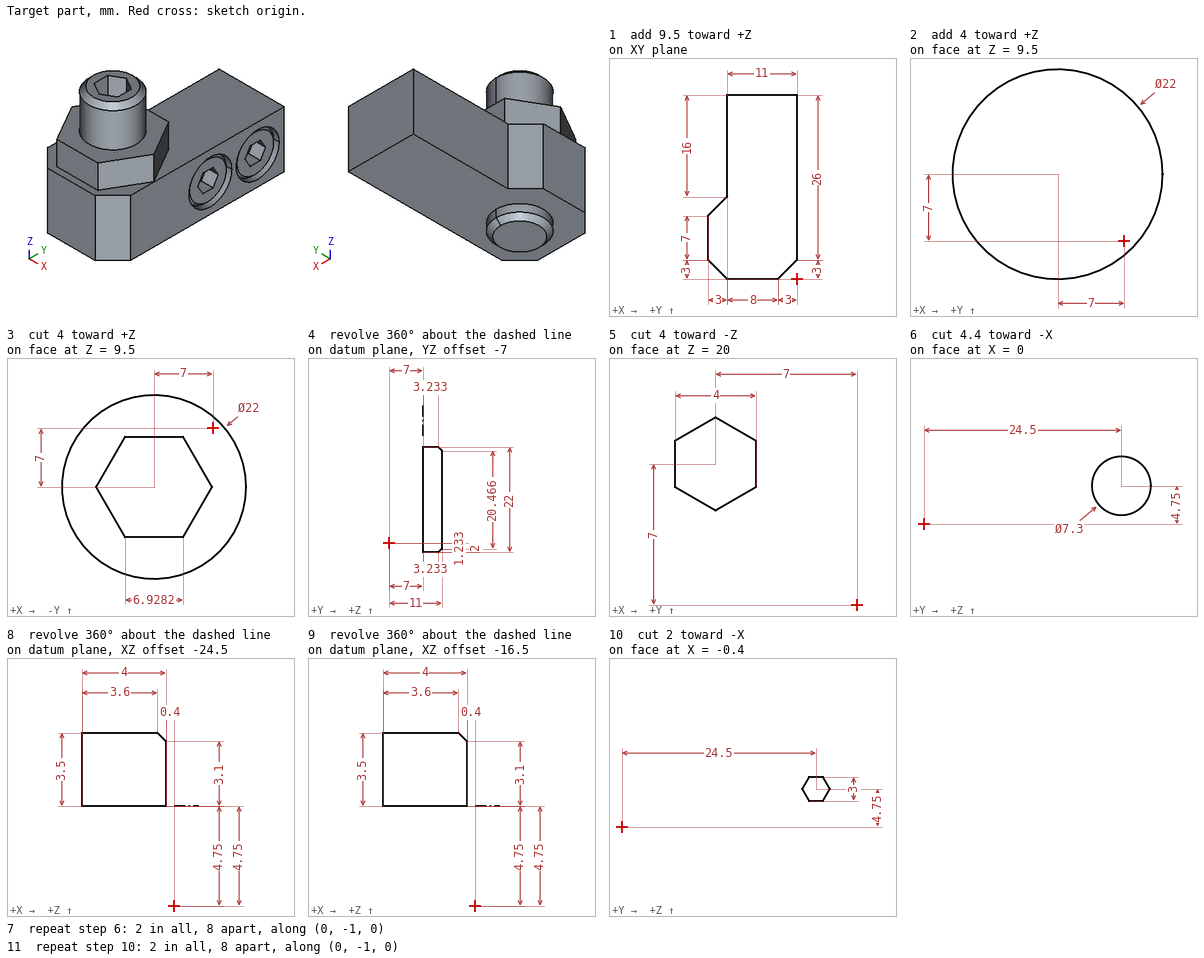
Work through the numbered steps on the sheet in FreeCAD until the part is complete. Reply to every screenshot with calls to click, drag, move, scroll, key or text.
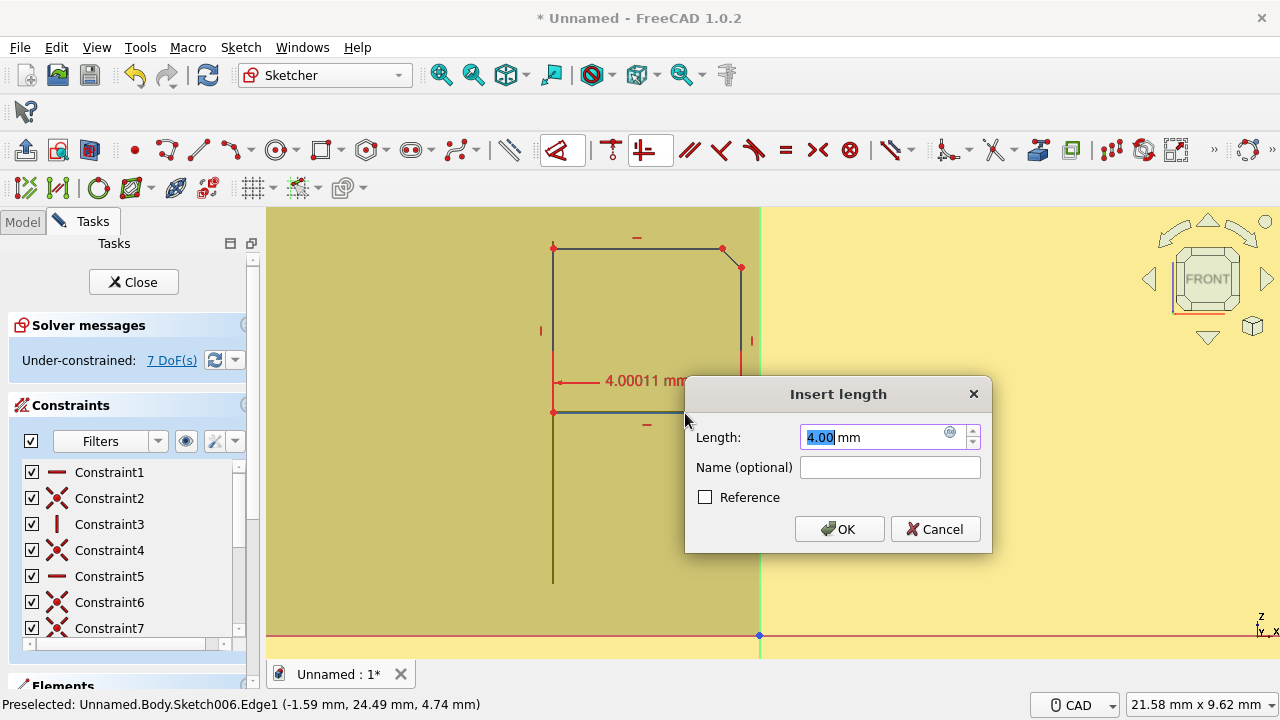
text(4)
key(Return)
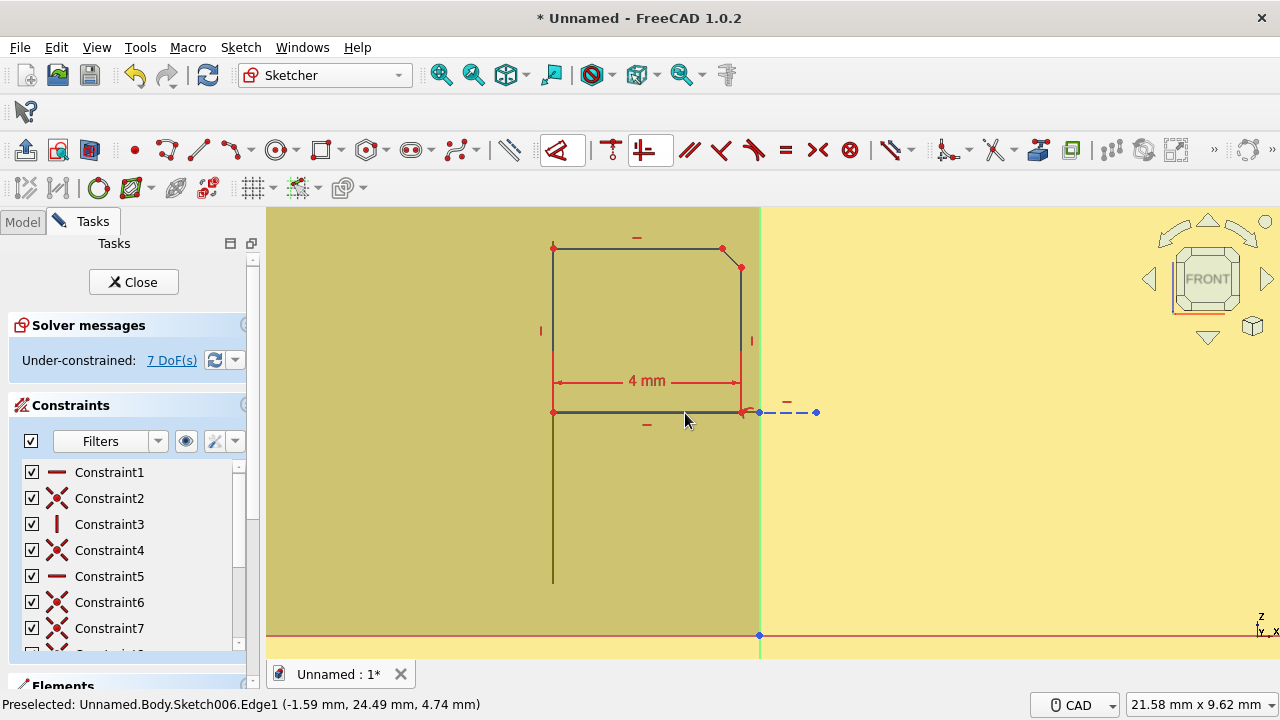
click(553, 364)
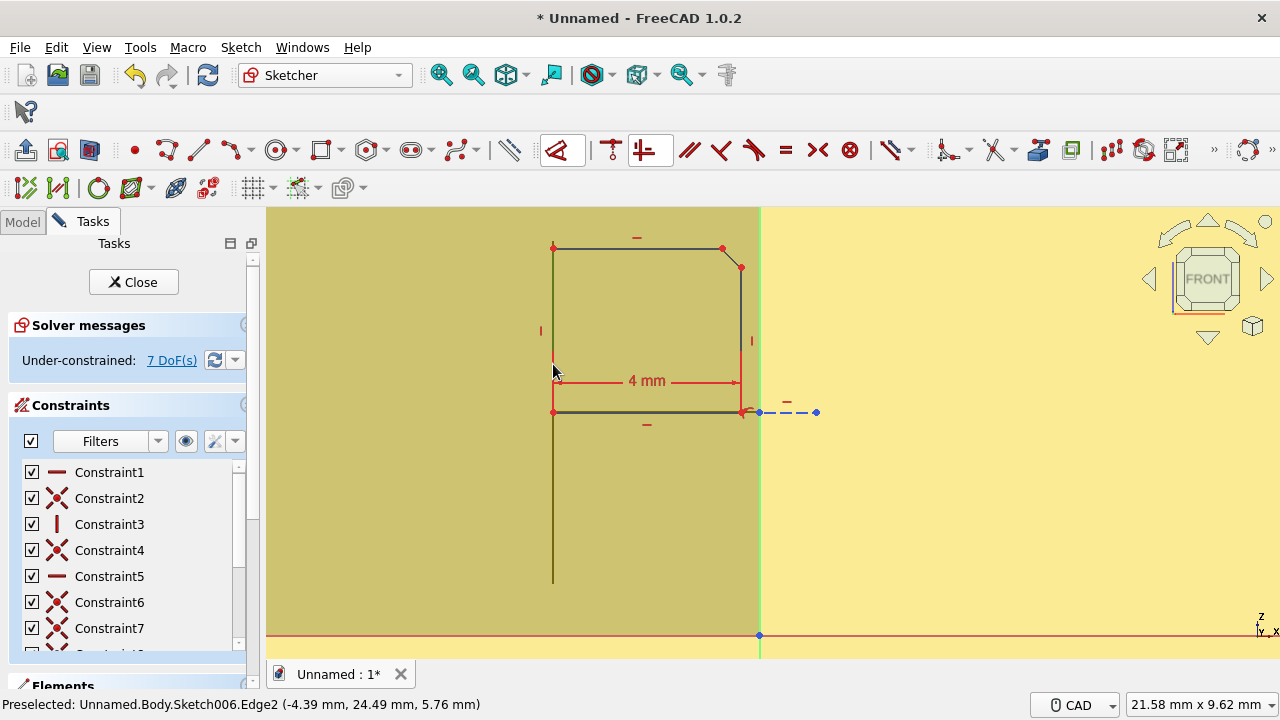
key(i)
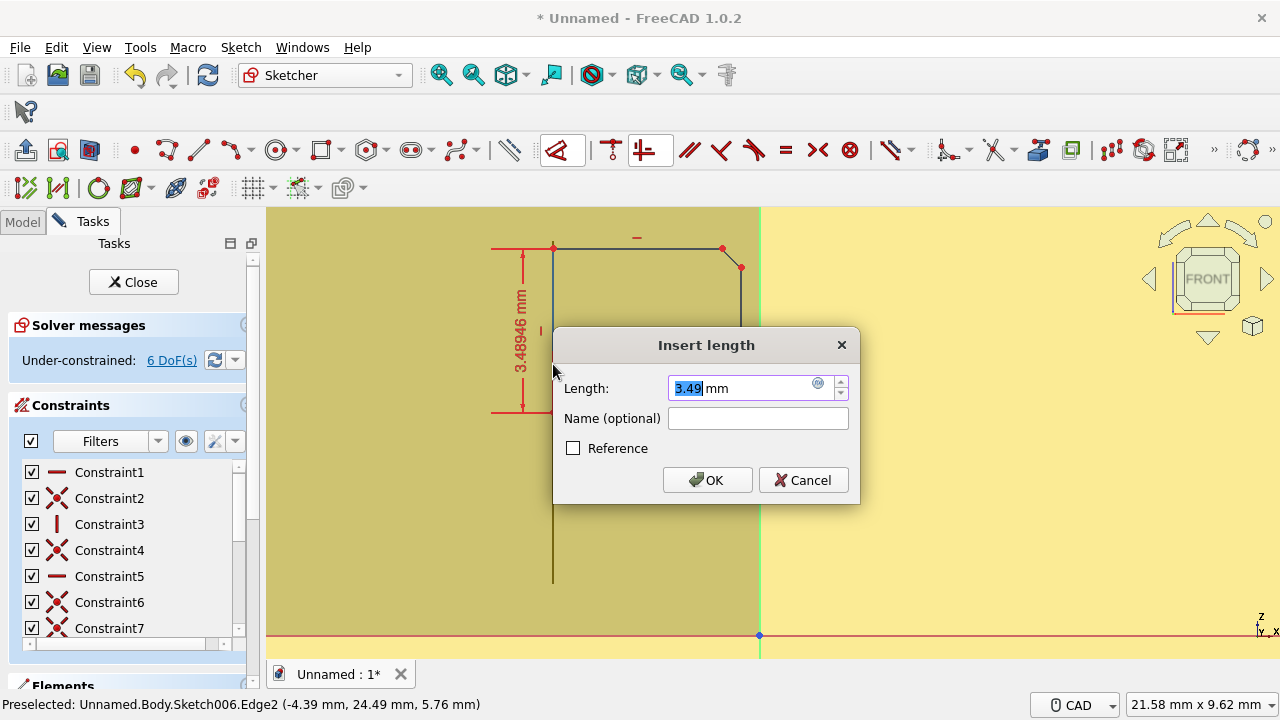
text(3.5)
key(Return)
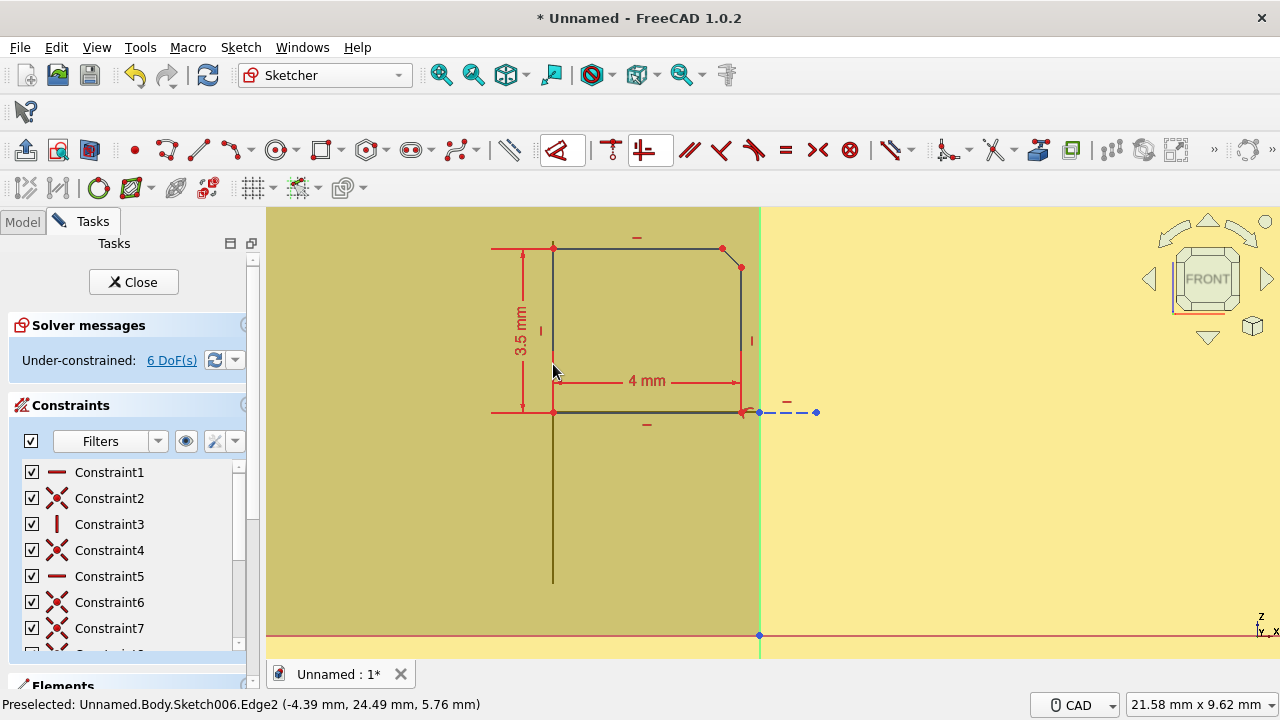
click(604, 249)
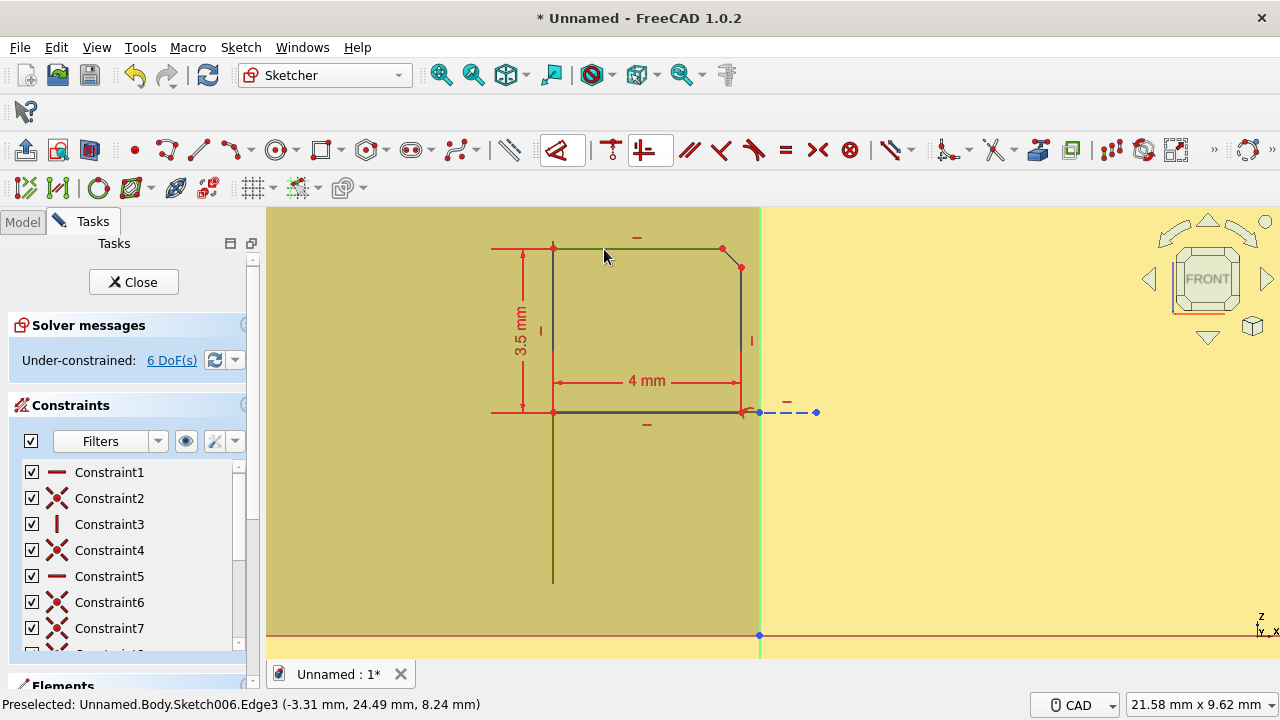
key(l)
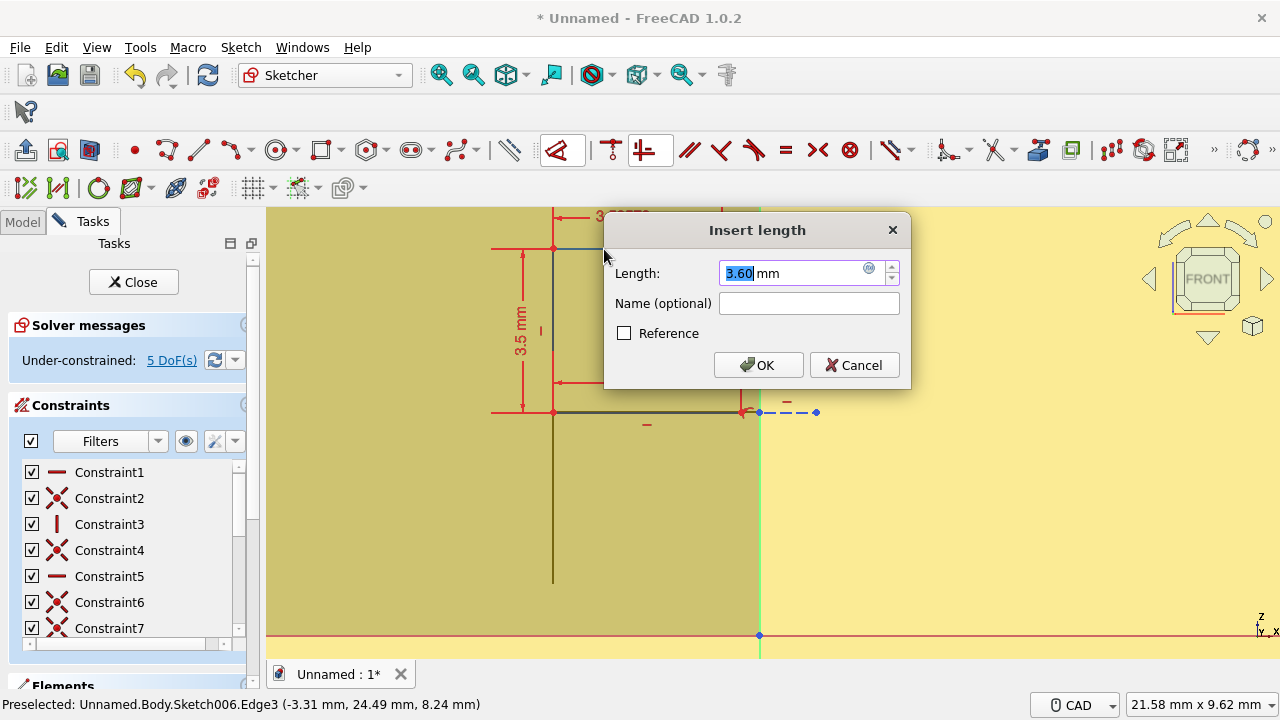
text(3.6)
key(Return)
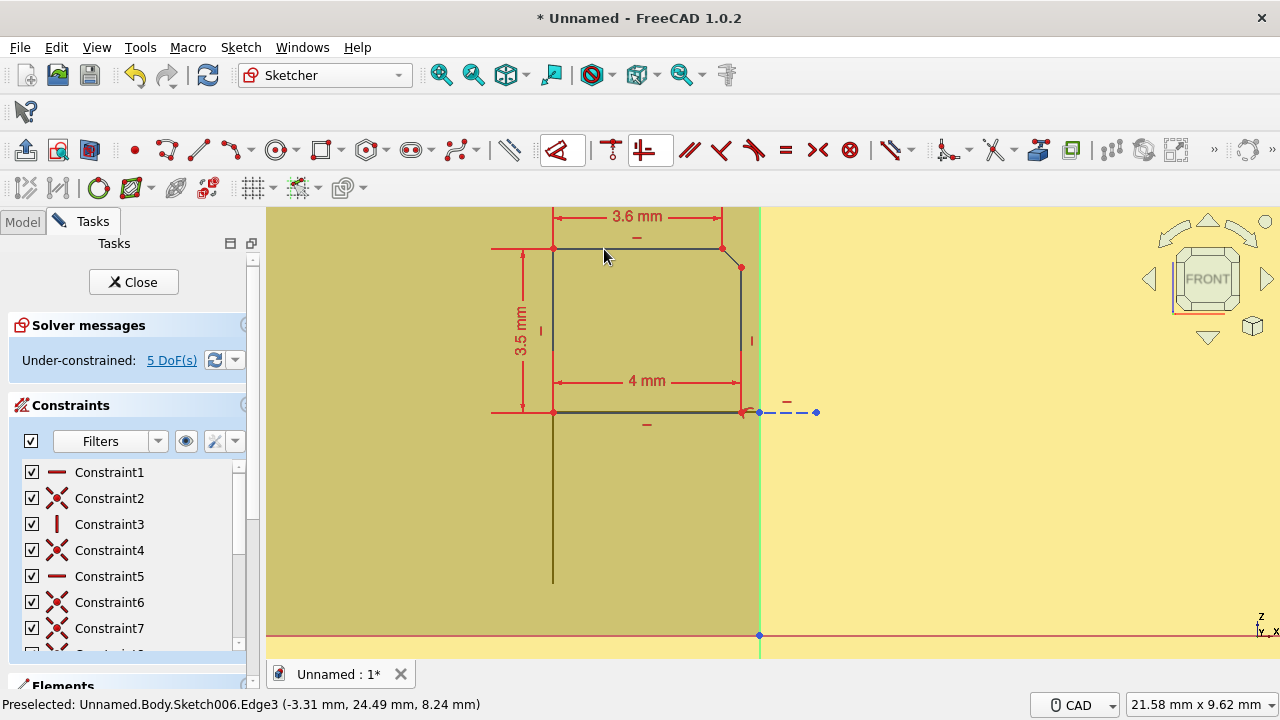
click(741, 312)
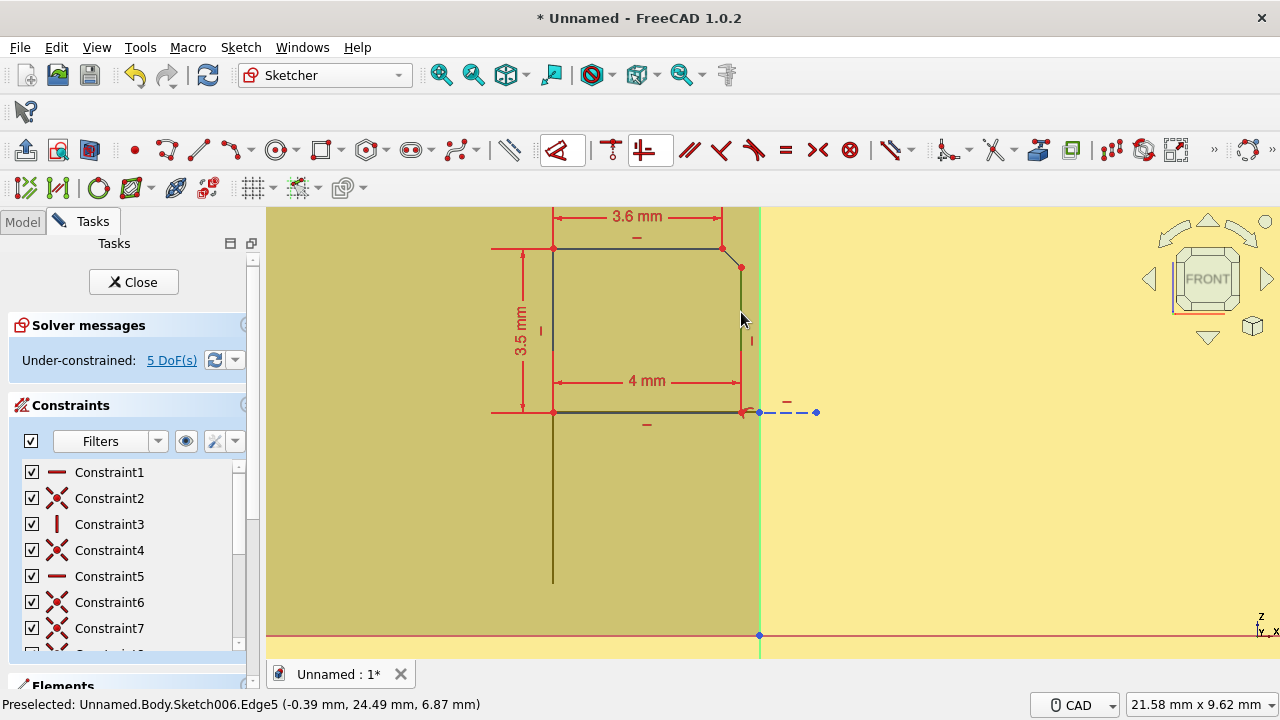
click(580, 150)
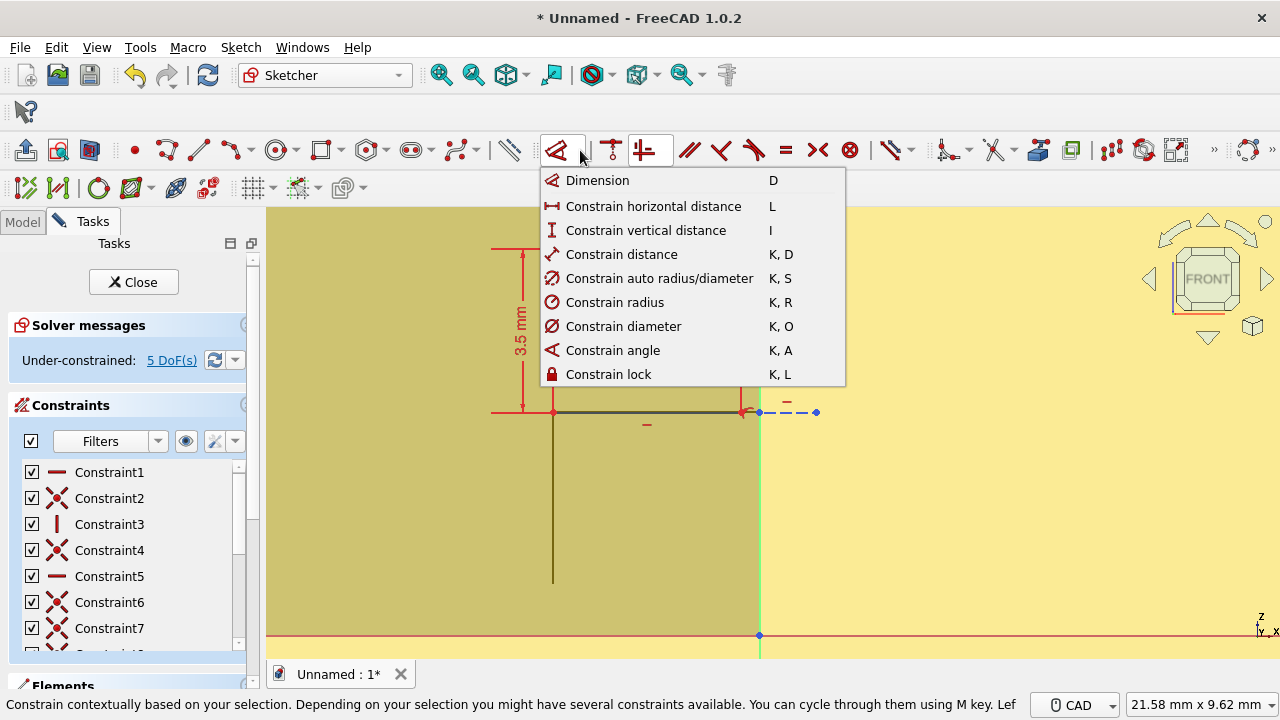
click(693, 230)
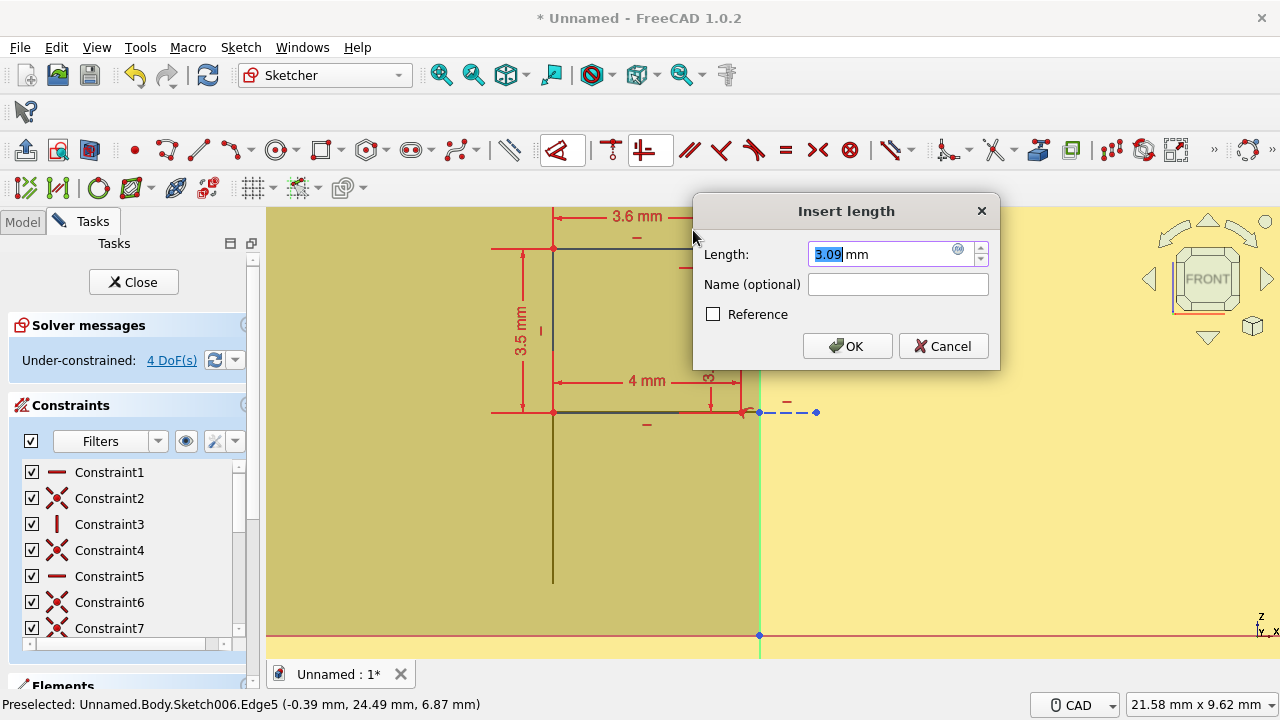
text(3.1)
key(Return)